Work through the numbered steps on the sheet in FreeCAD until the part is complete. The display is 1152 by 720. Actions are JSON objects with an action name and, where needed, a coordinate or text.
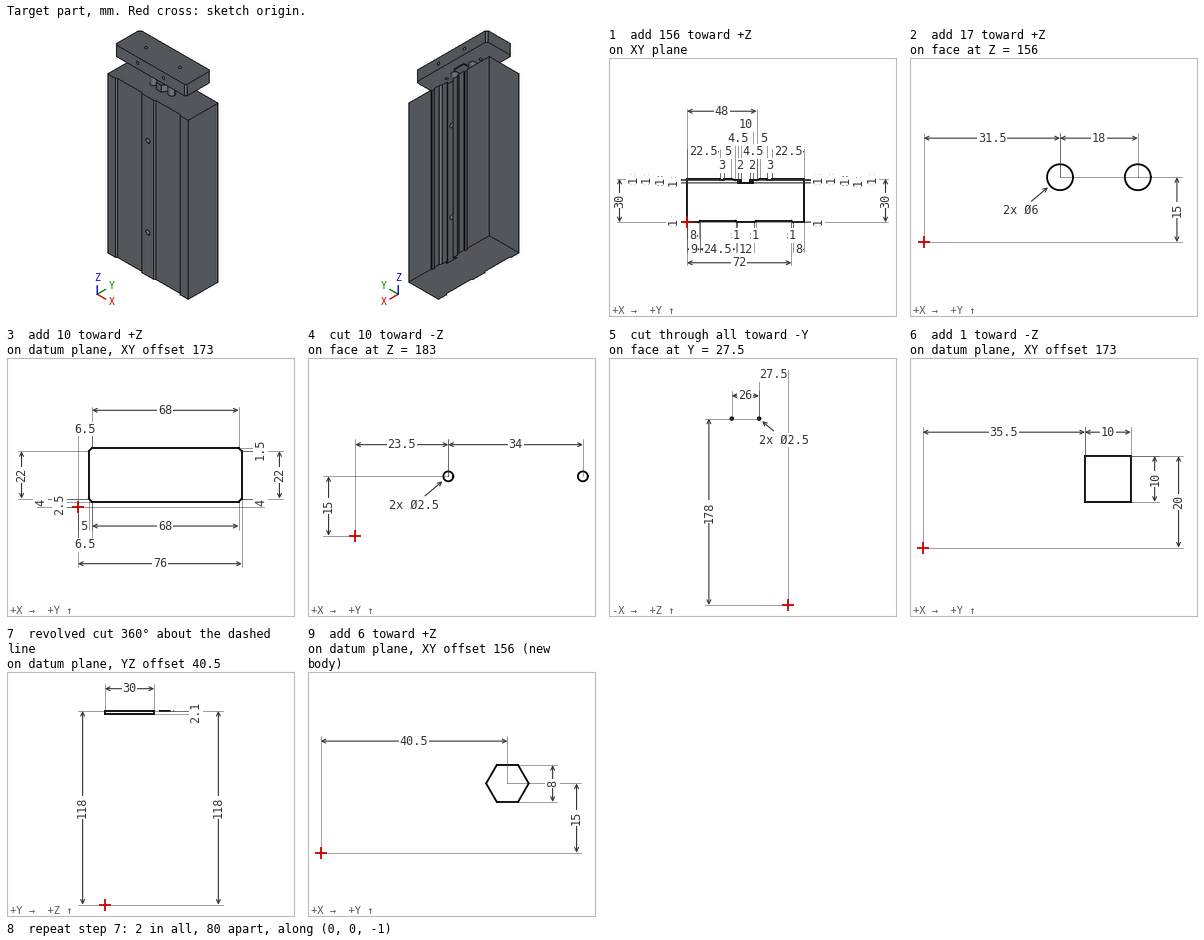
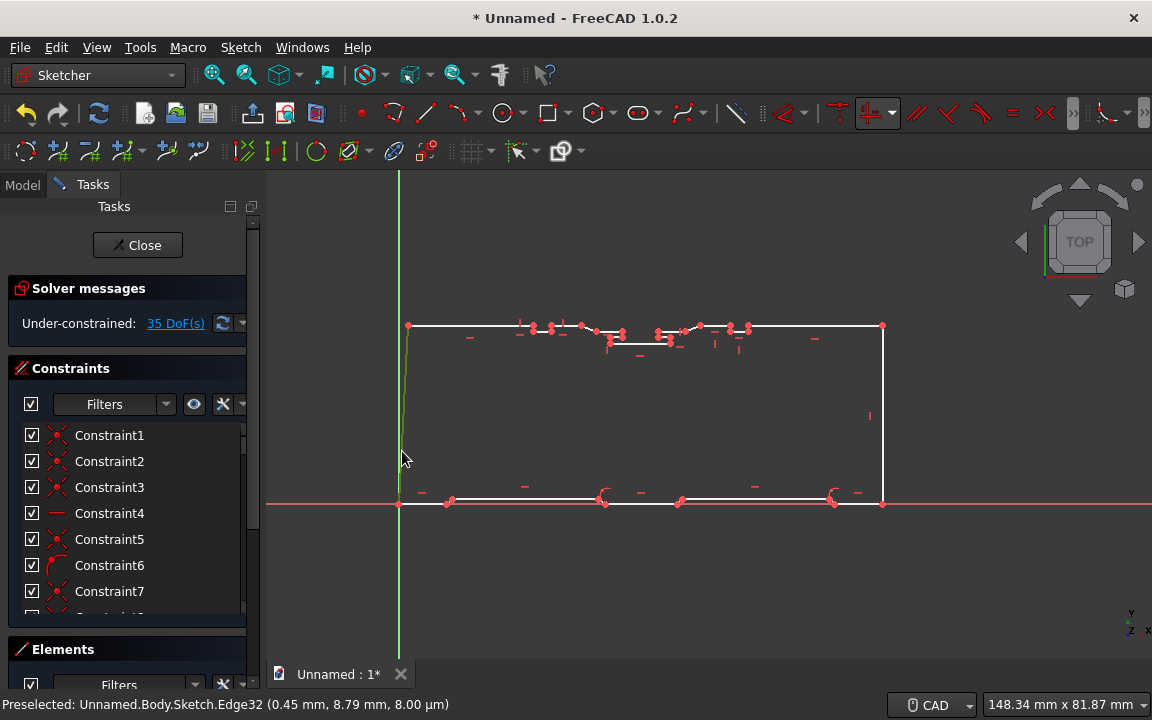
{"action": "key", "text": "v"}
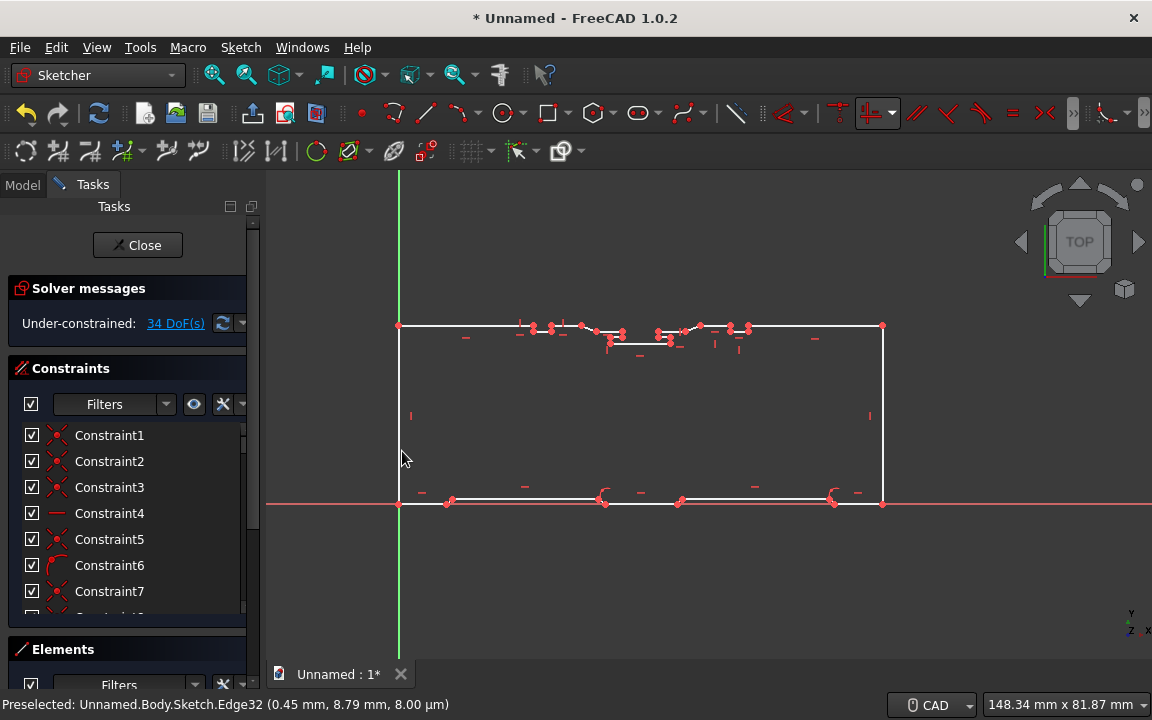
{"action": "left_click", "coordinate": [784, 114]}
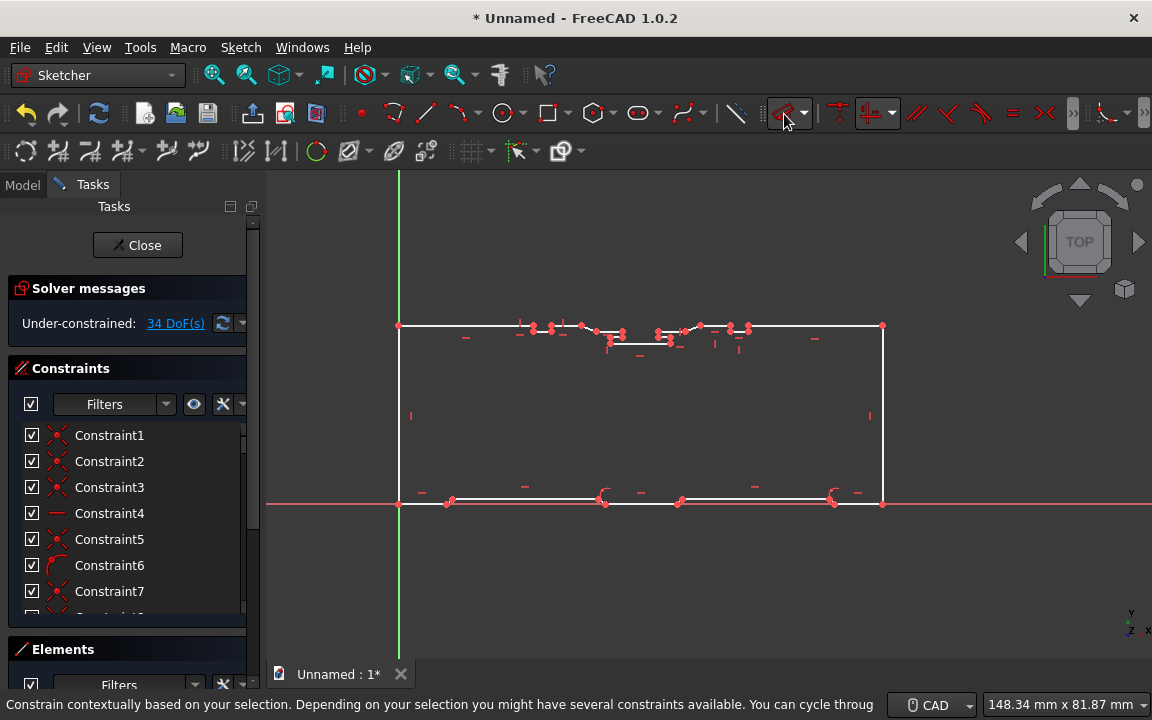
{"action": "left_click", "coordinate": [413, 504]}
{"action": "left_click", "coordinate": [423, 538]}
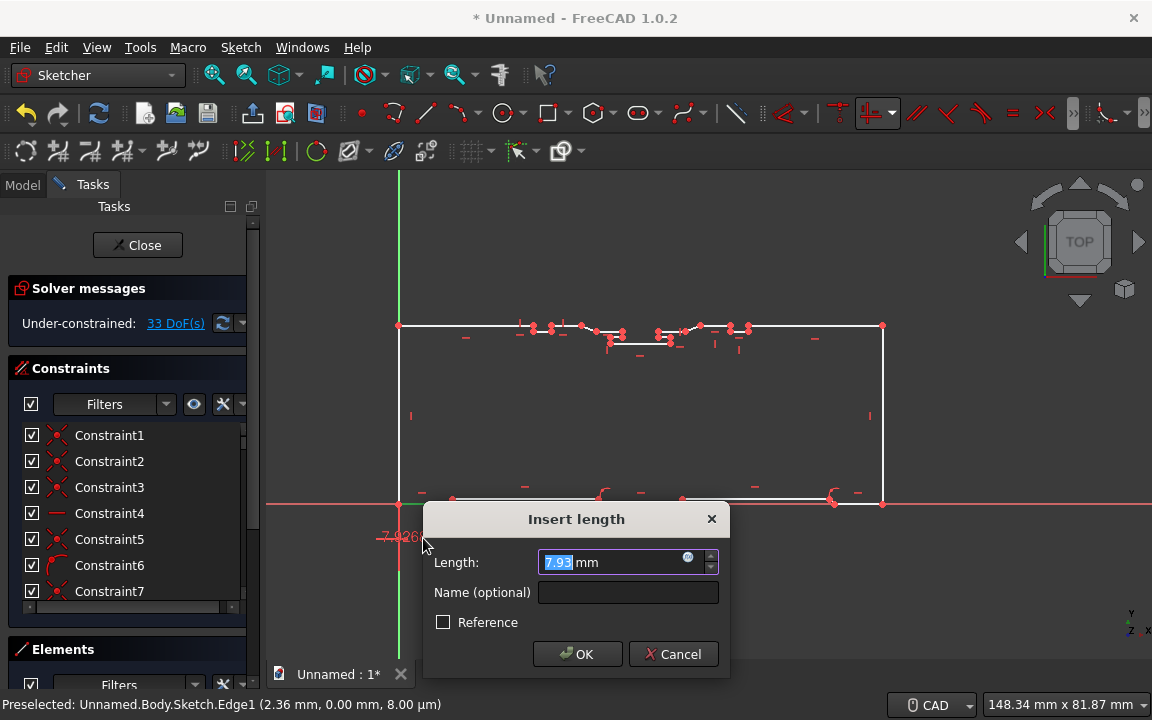
{"action": "type", "text": "8"}
{"action": "key", "text": "Return"}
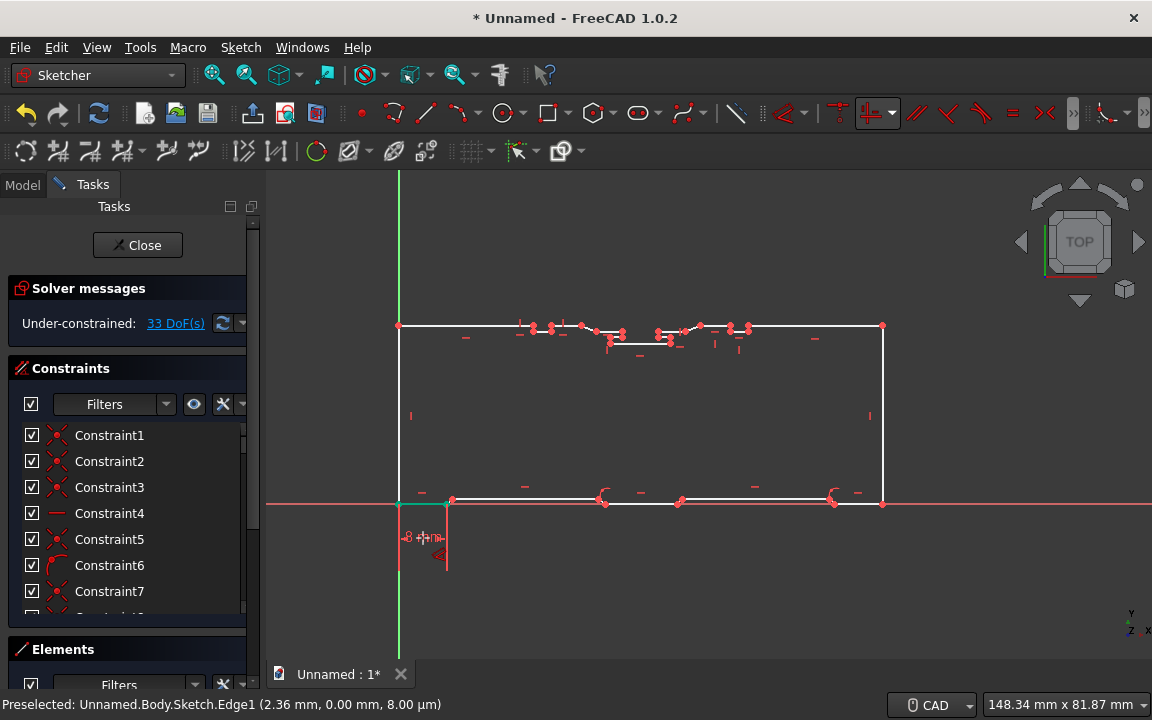
{"action": "left_click", "coordinate": [849, 504]}
{"action": "left_click", "coordinate": [859, 538]}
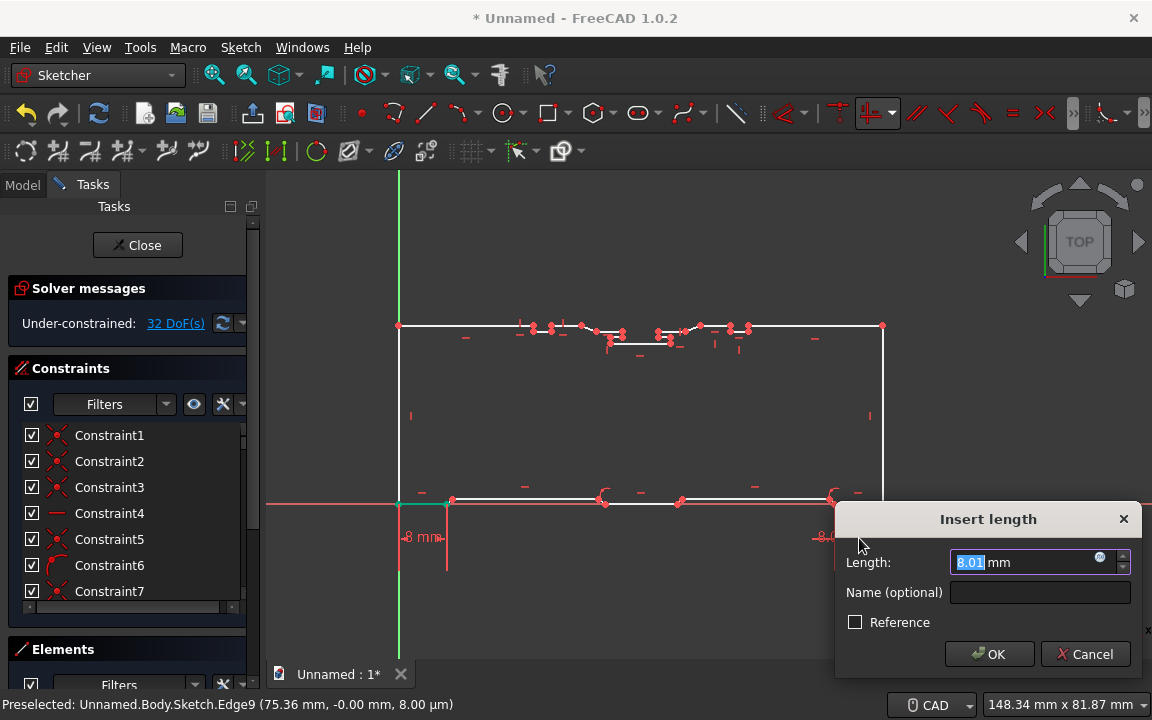
{"action": "type", "text": "8"}
{"action": "key", "text": "Return"}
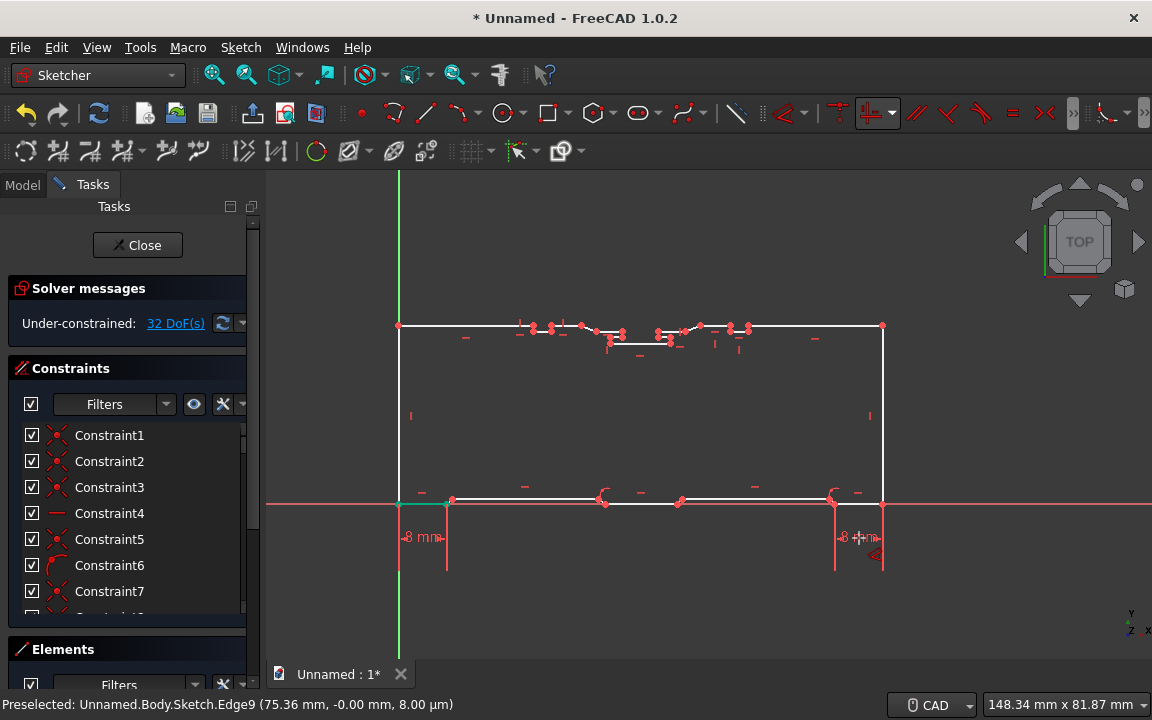
{"action": "scroll", "coordinate": [748, 329], "scroll_direction": "up", "scroll_amount": 10}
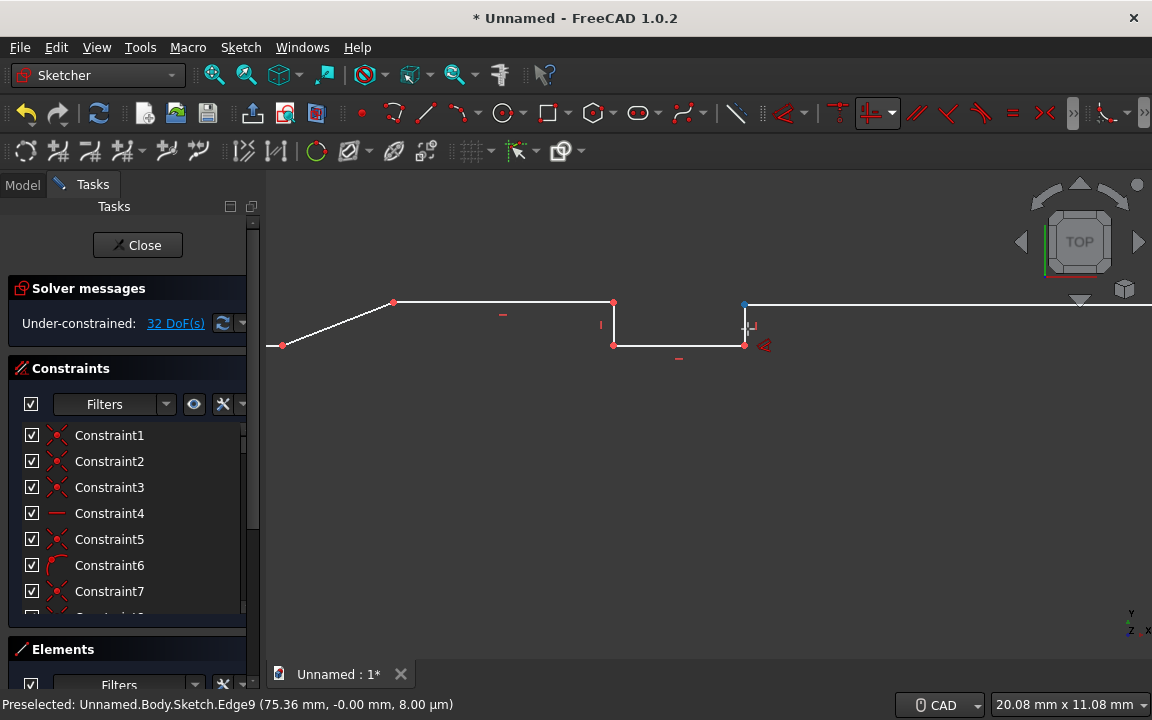
{"action": "left_click", "coordinate": [745, 325]}
{"action": "left_click", "coordinate": [779, 325]}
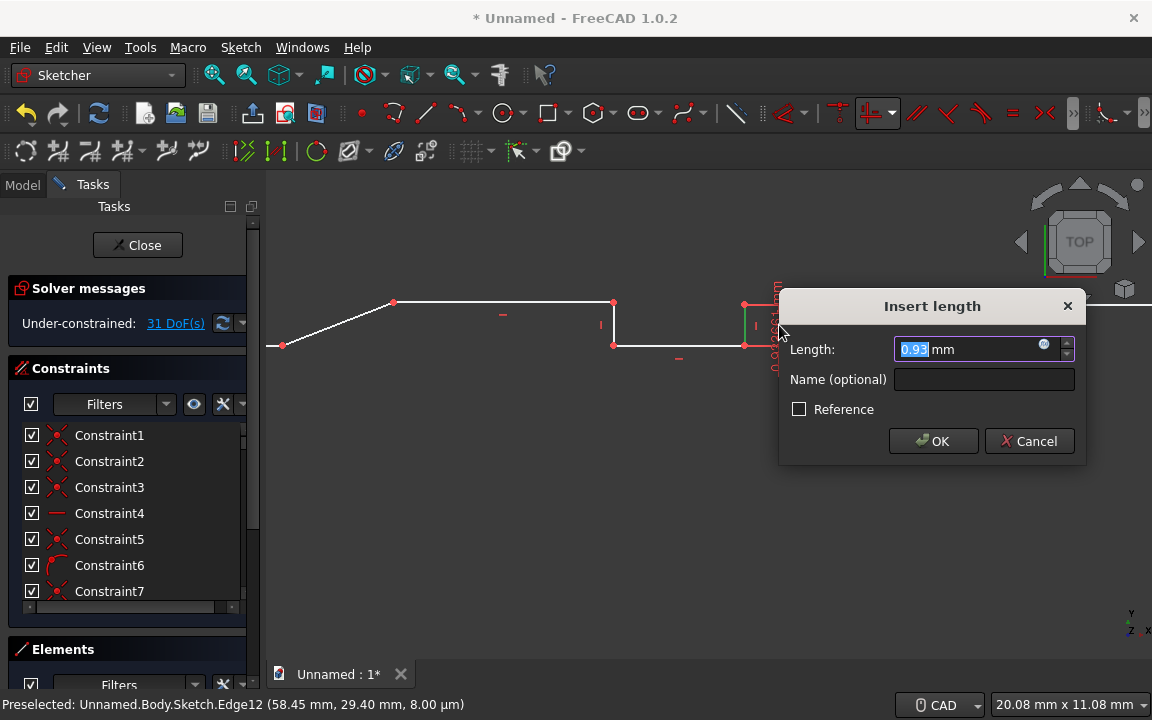
{"action": "type", "text": "1"}
{"action": "key", "text": "Return"}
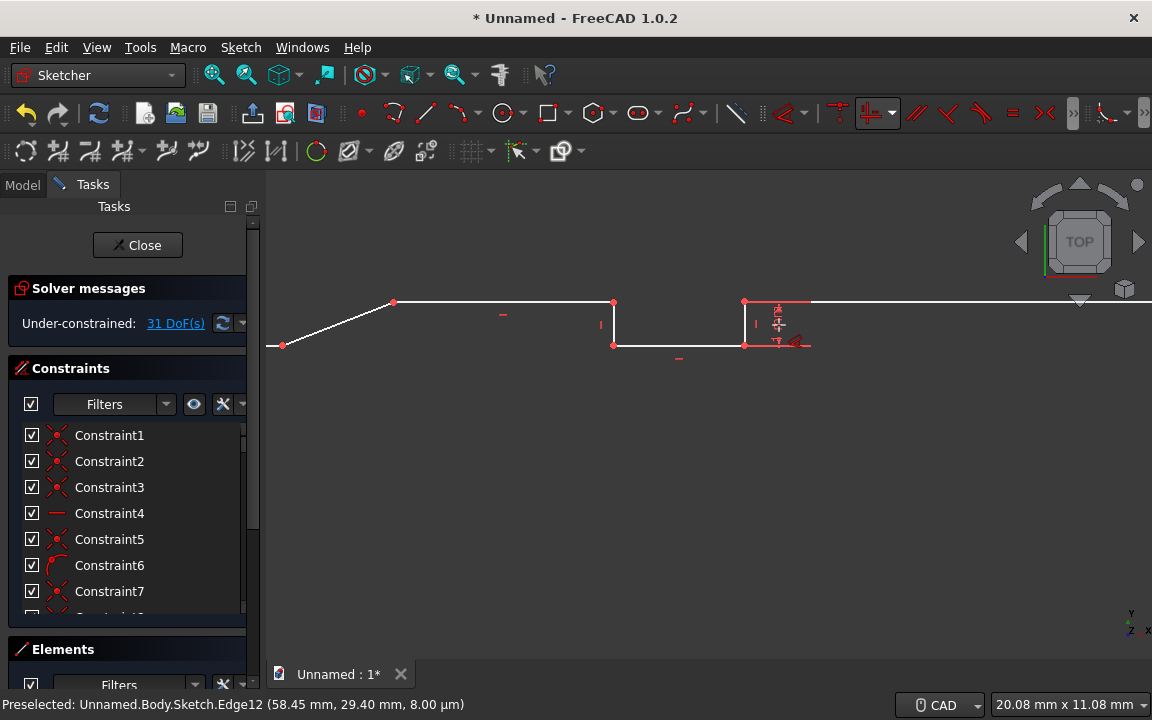
{"action": "left_click", "coordinate": [705, 346]}
{"action": "left_click", "coordinate": [679, 312]}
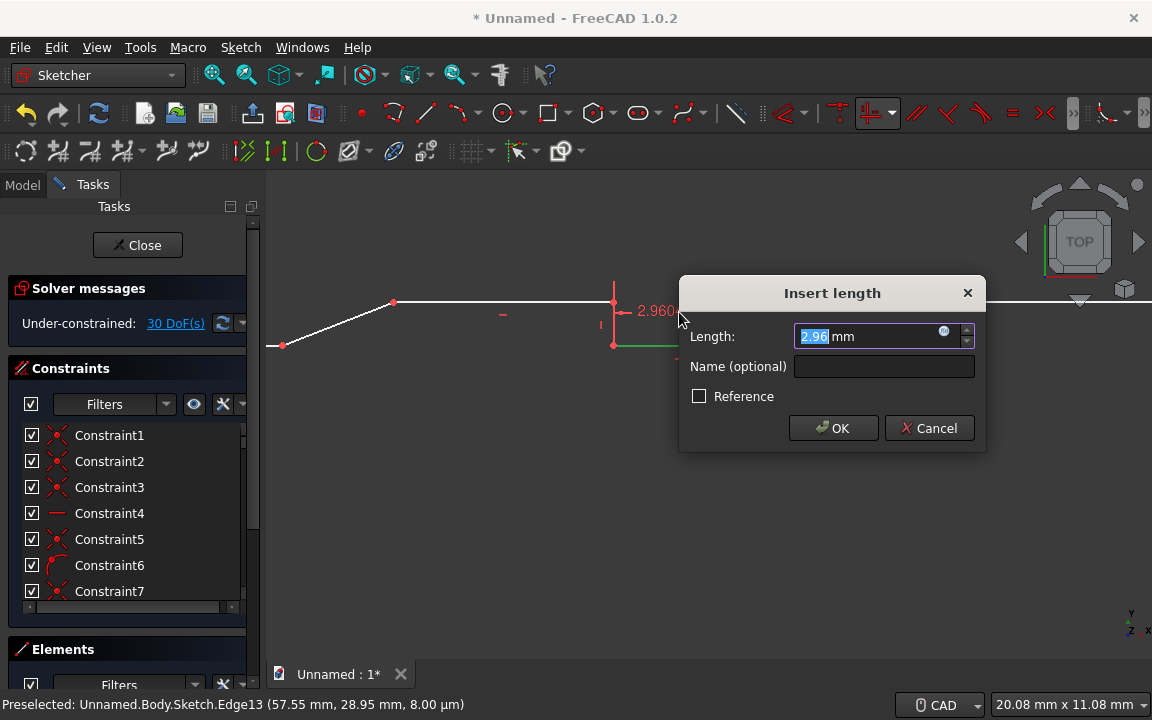
{"action": "type", "text": "3"}
{"action": "key", "text": "Return"}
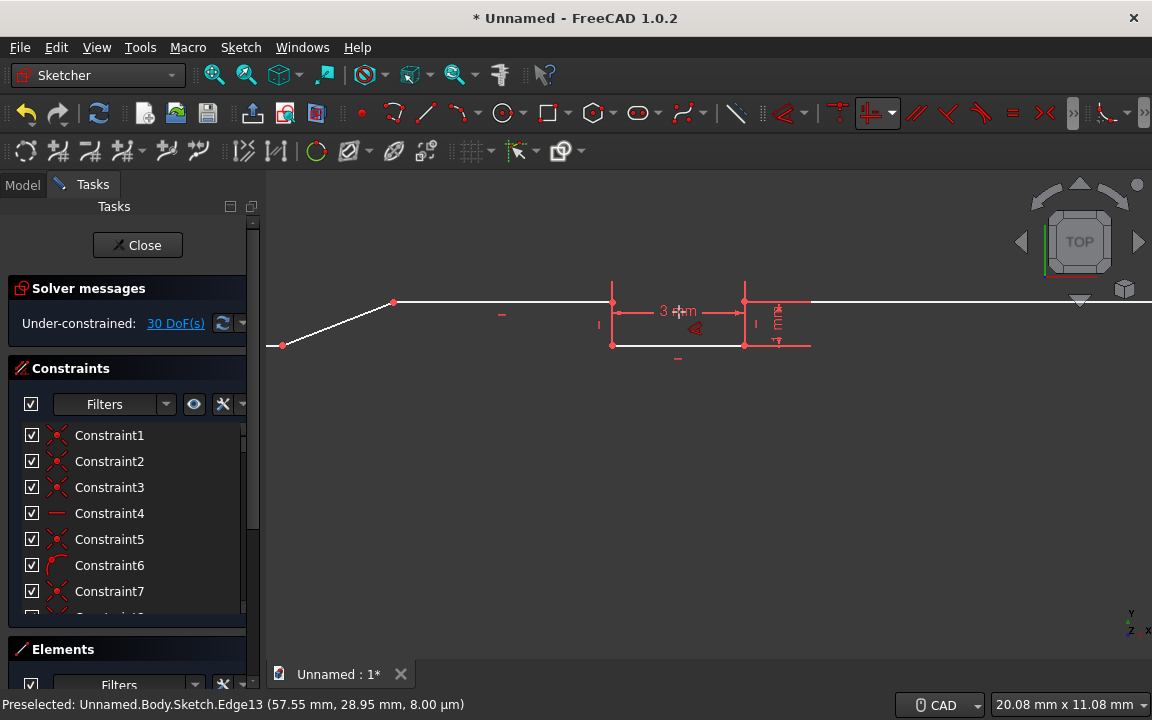
{"action": "left_click", "coordinate": [612, 333]}
{"action": "left_click", "coordinate": [578, 324]}